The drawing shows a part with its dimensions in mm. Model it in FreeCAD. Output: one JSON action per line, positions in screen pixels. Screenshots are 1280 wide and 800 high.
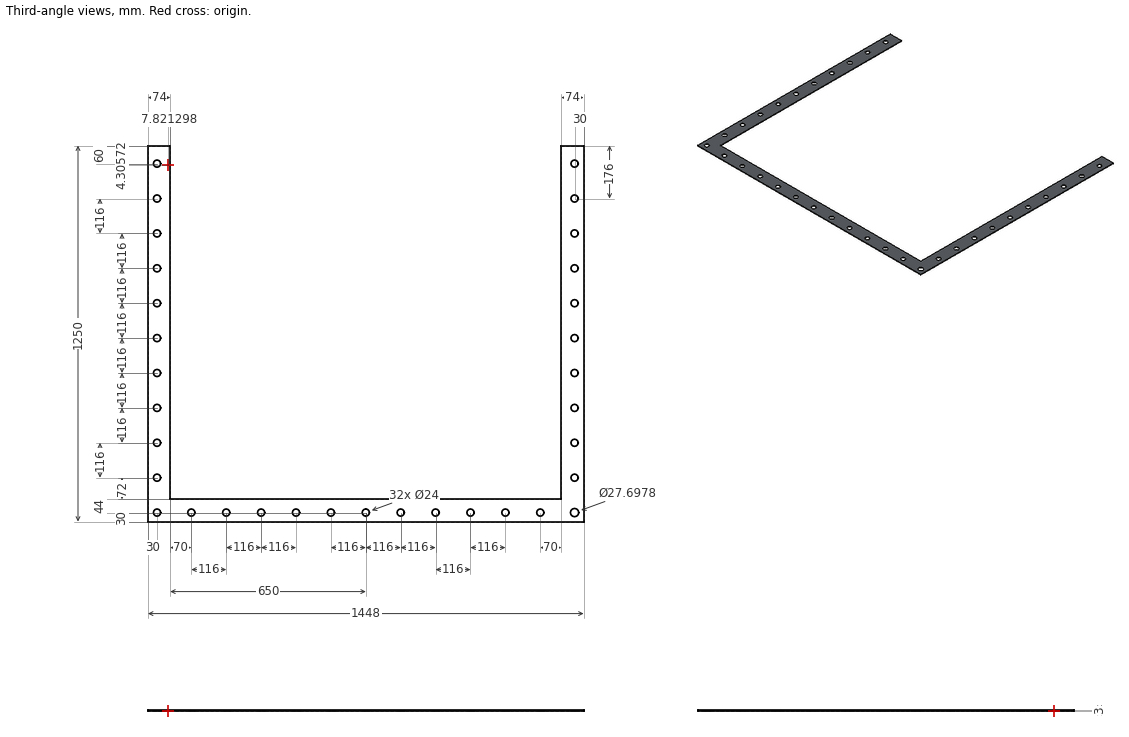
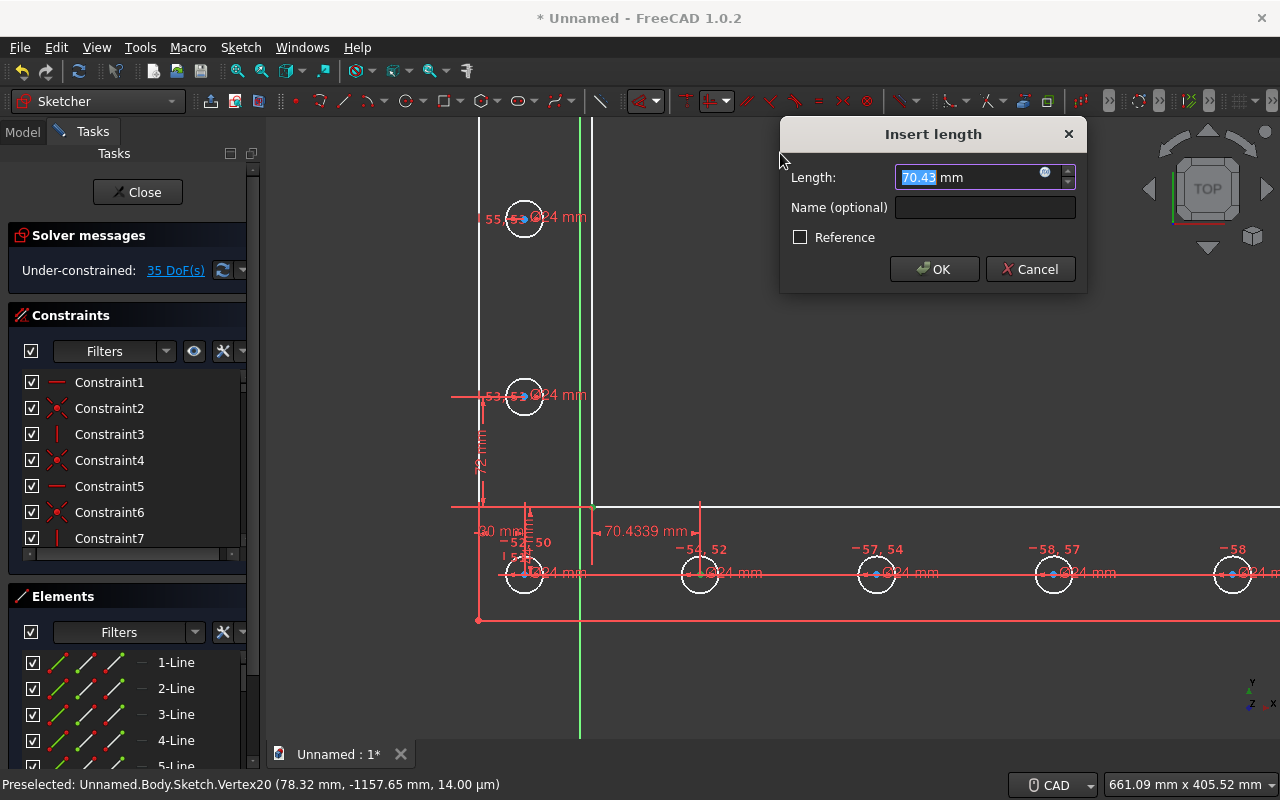
{"action": "type", "text": "70"}
{"action": "key", "text": "Return"}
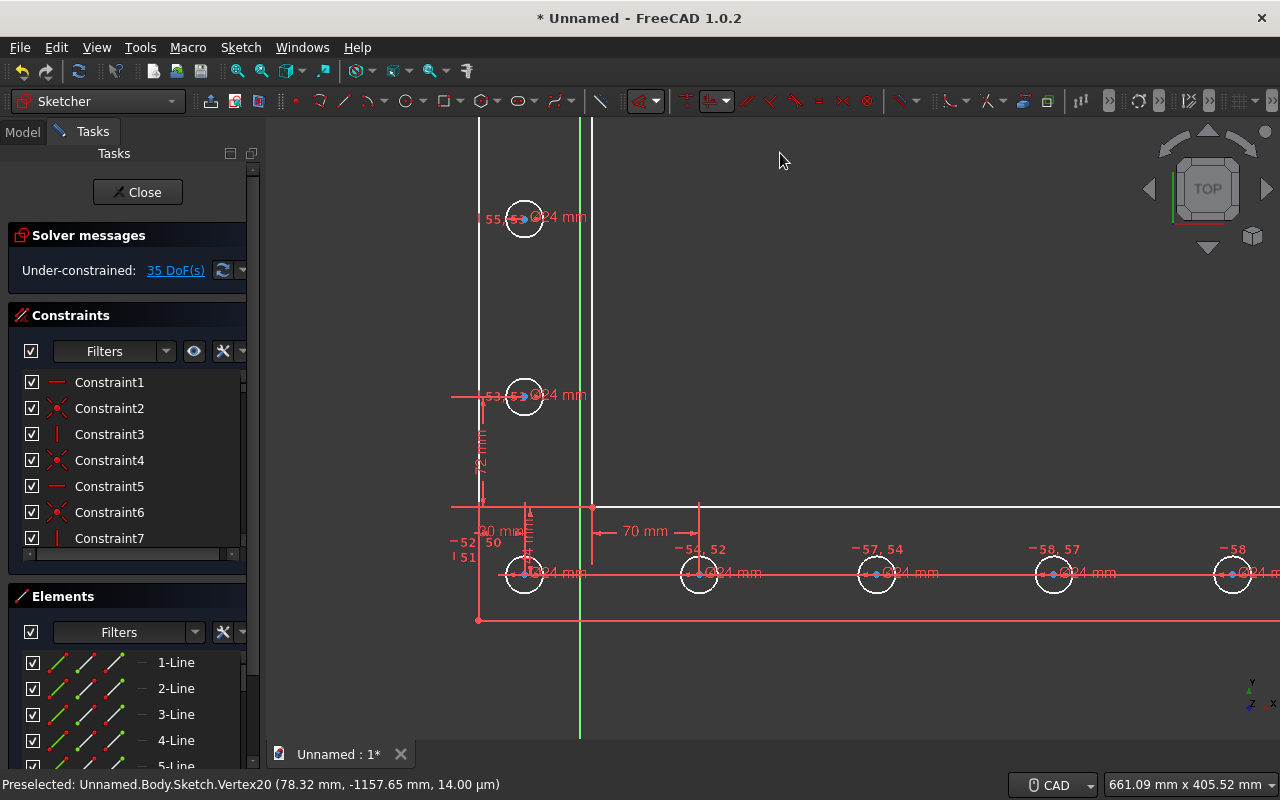
{"action": "scroll", "coordinate": [481, 622], "scroll_direction": "down", "scroll_amount": 8}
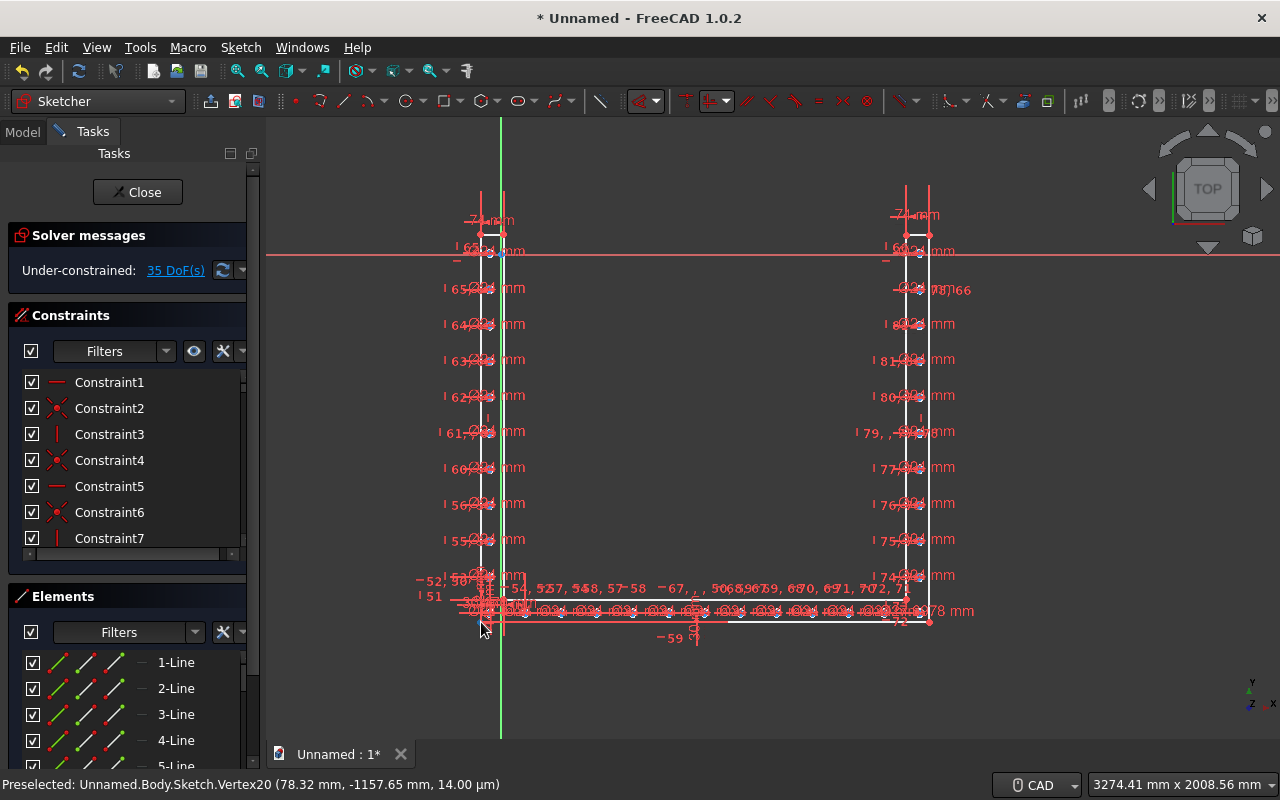
{"action": "scroll", "coordinate": [481, 235], "scroll_direction": "up", "scroll_amount": 4}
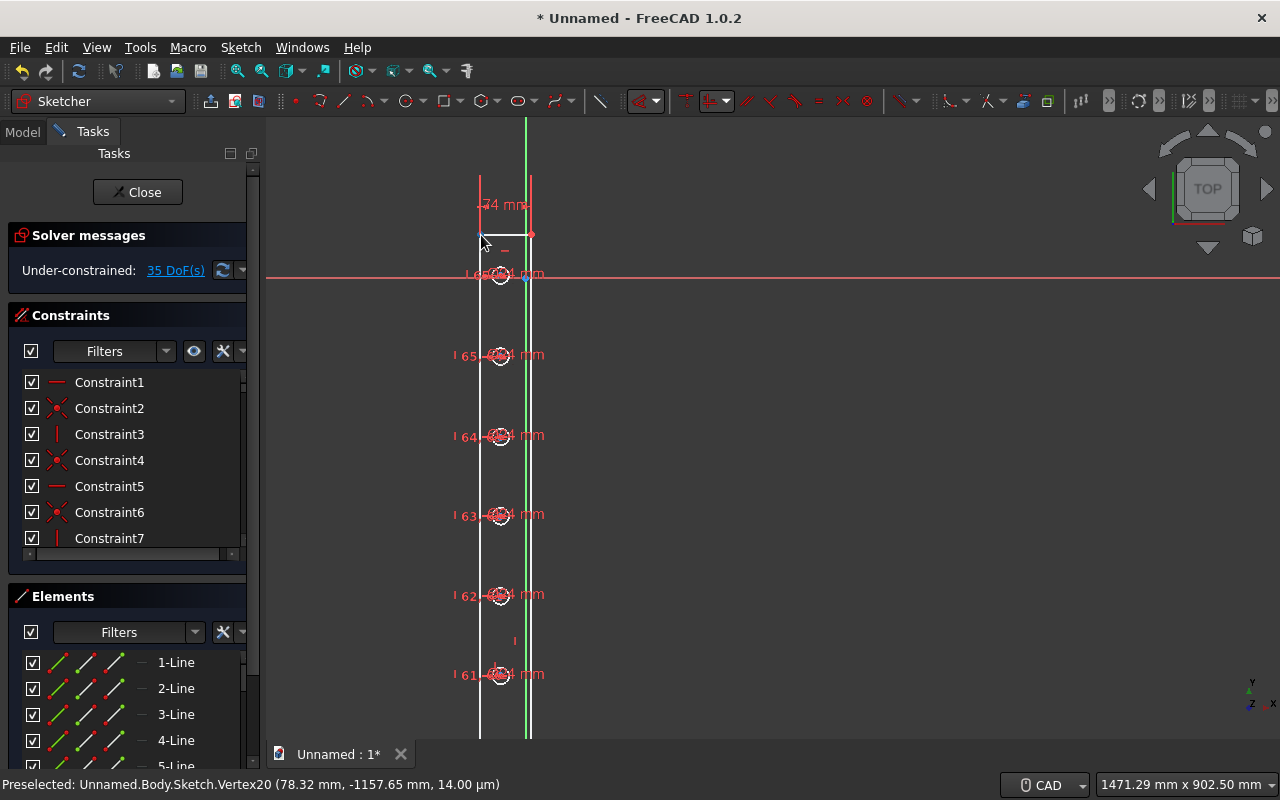
{"action": "left_click", "coordinate": [480, 235]}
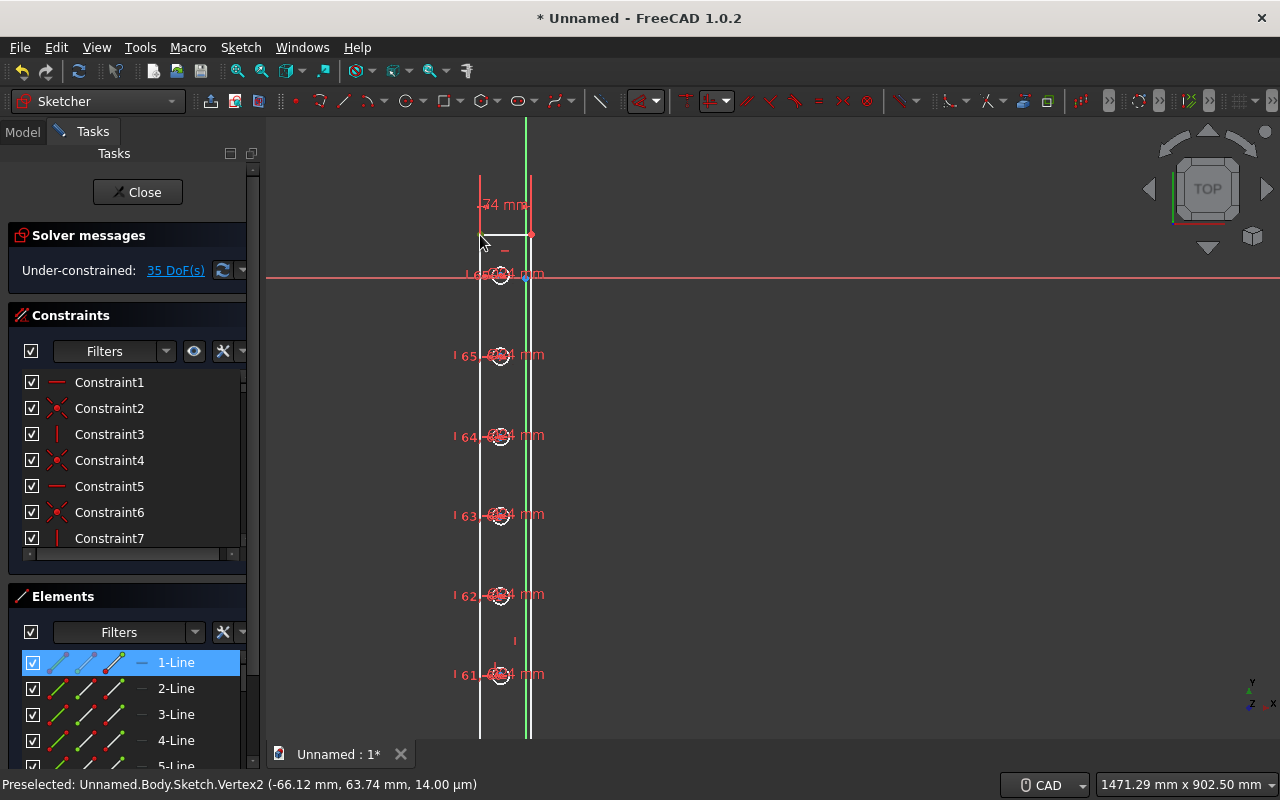
{"action": "left_click", "coordinate": [501, 276]}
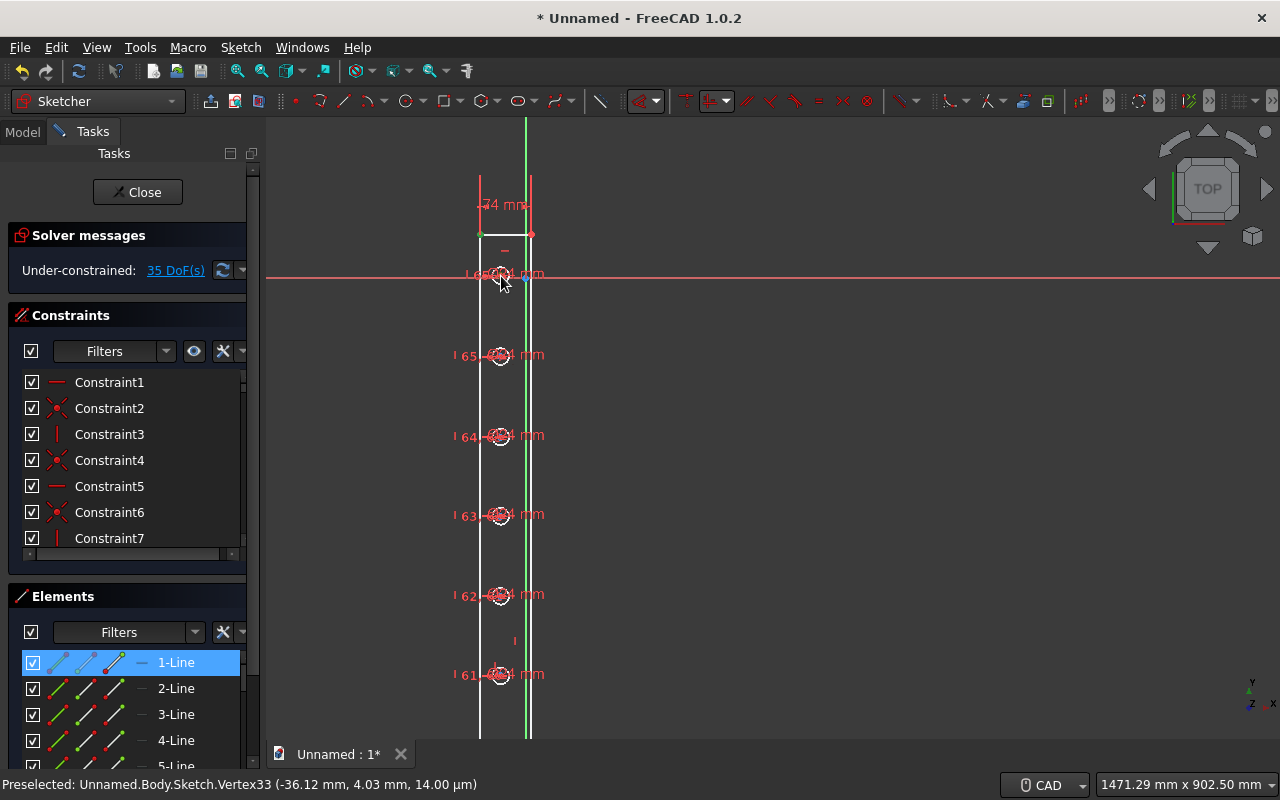
{"action": "key", "text": "i"}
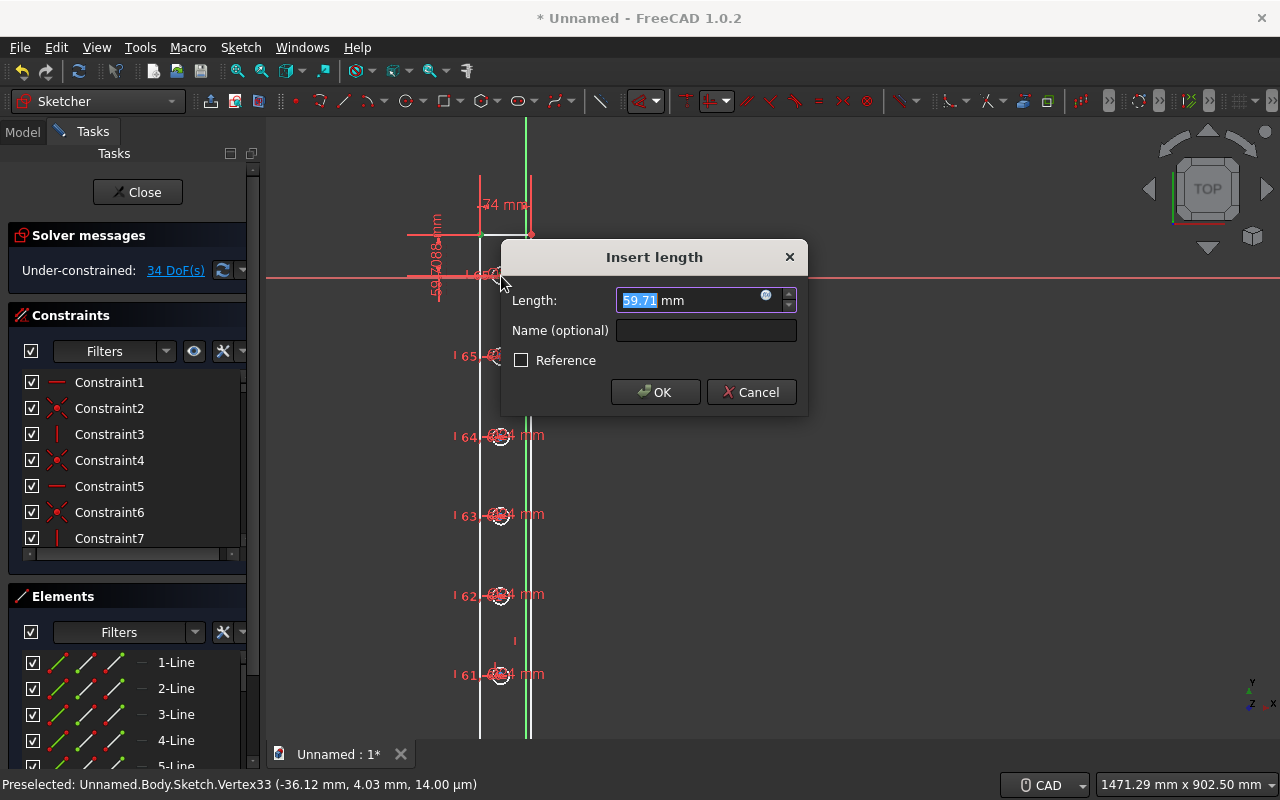
{"action": "type", "text": "60"}
{"action": "key", "text": "Return"}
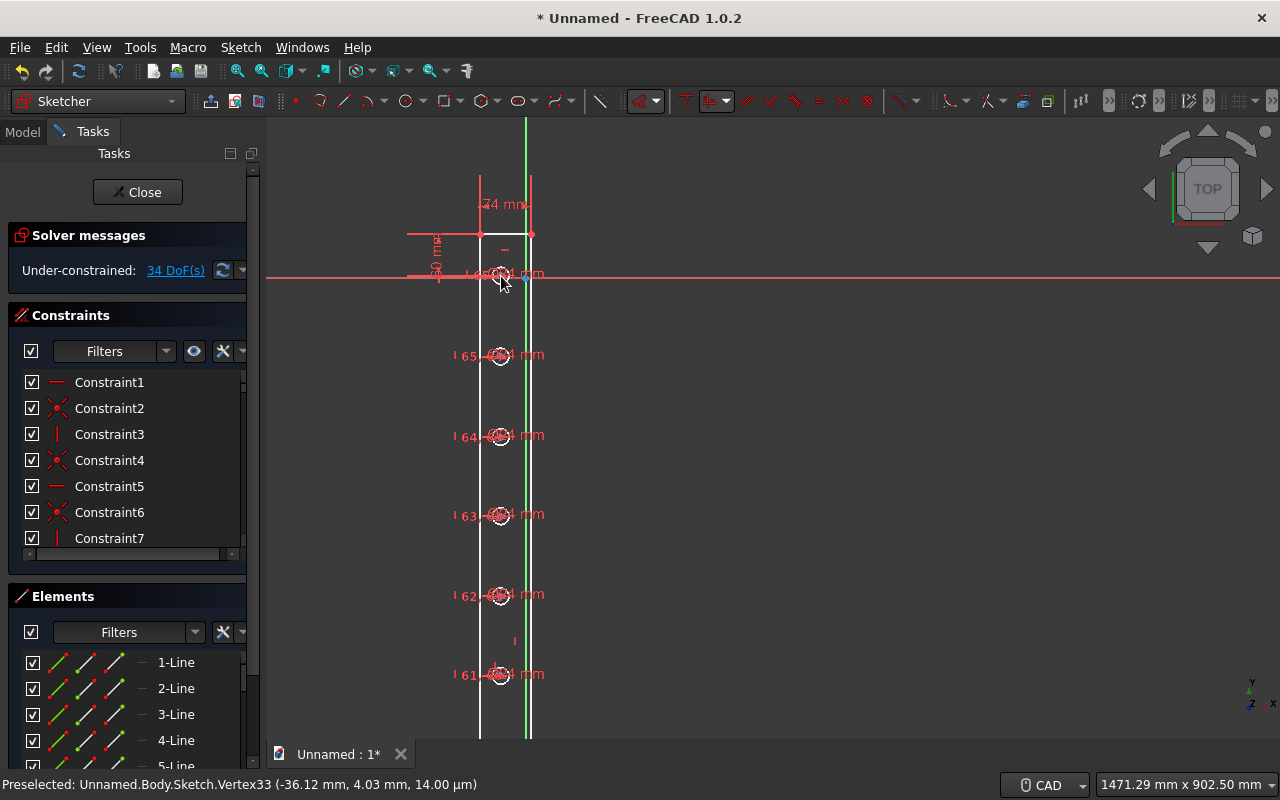
{"action": "scroll", "coordinate": [481, 235], "scroll_direction": "down", "scroll_amount": 4}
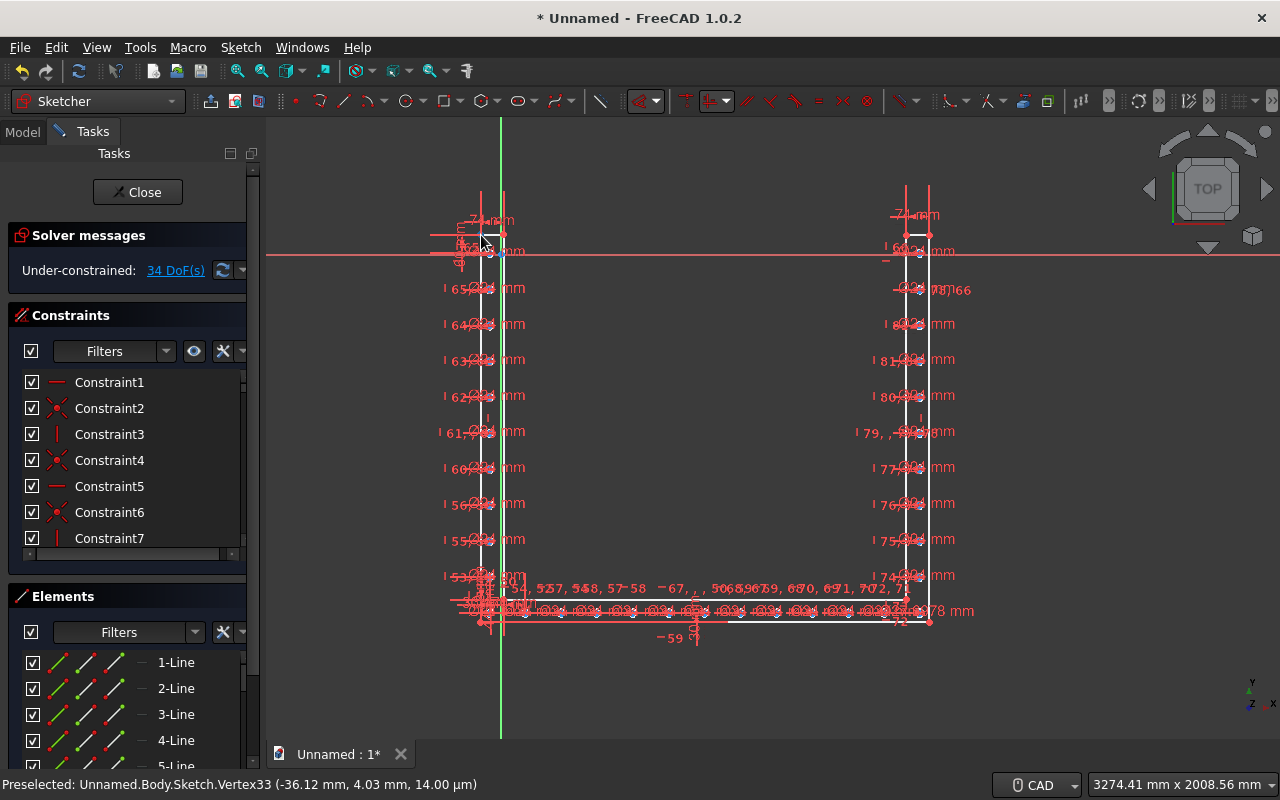
{"action": "scroll", "coordinate": [929, 235], "scroll_direction": "up", "scroll_amount": 8}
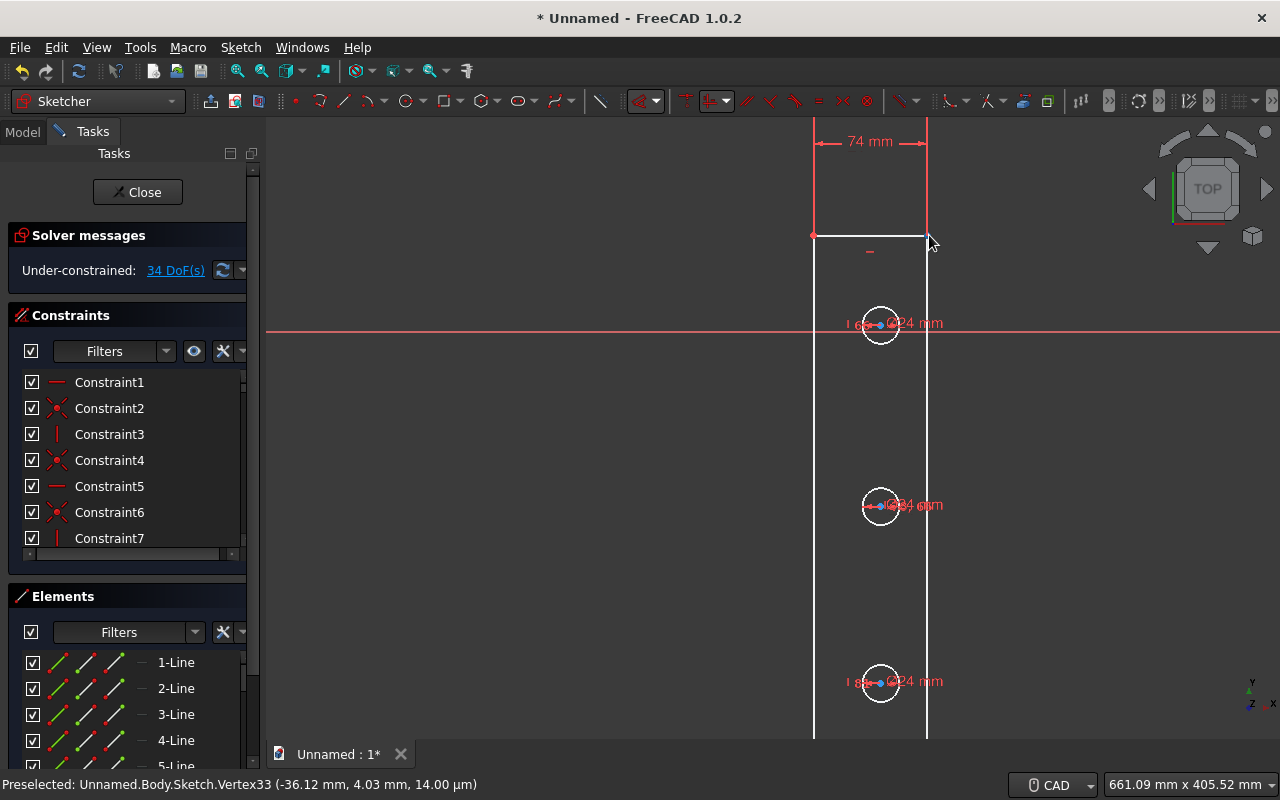
{"action": "left_click", "coordinate": [927, 236]}